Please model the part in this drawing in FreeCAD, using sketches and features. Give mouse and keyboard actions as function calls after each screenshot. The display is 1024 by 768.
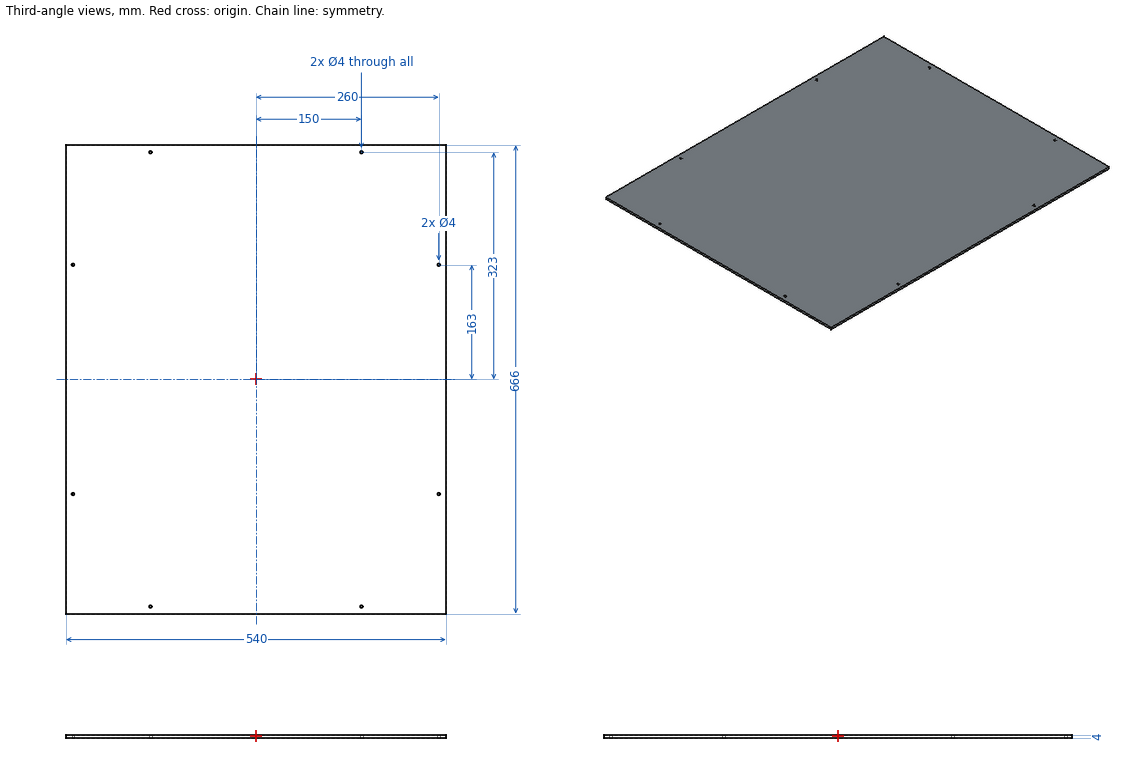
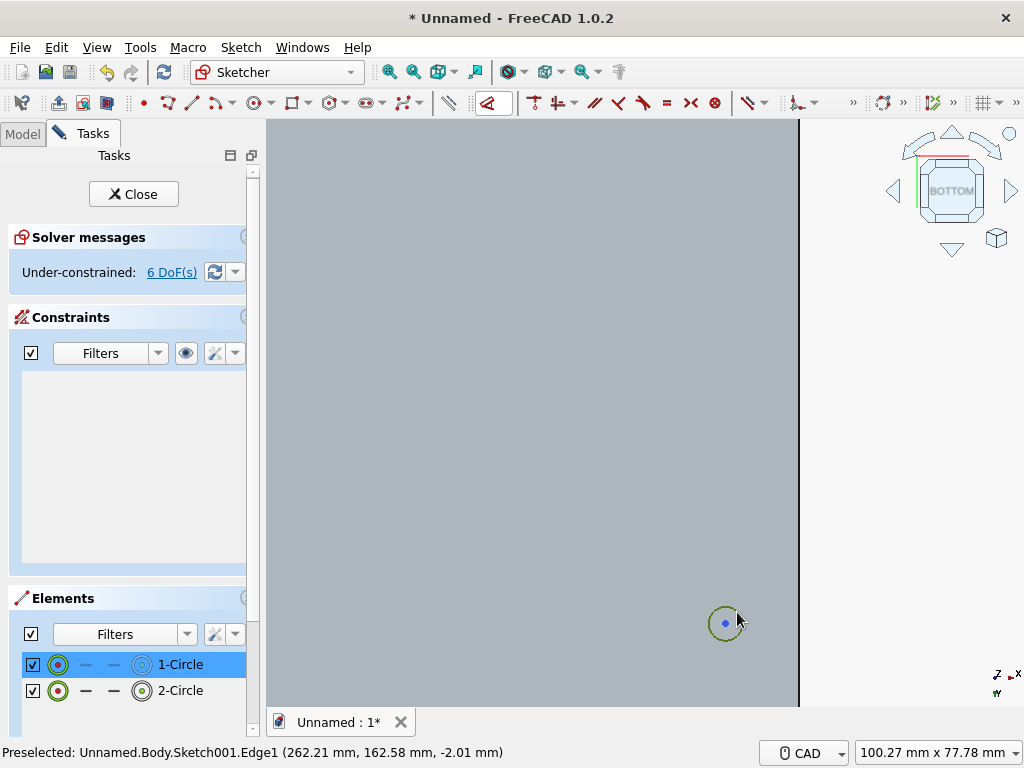
scroll(740, 616, down, 9)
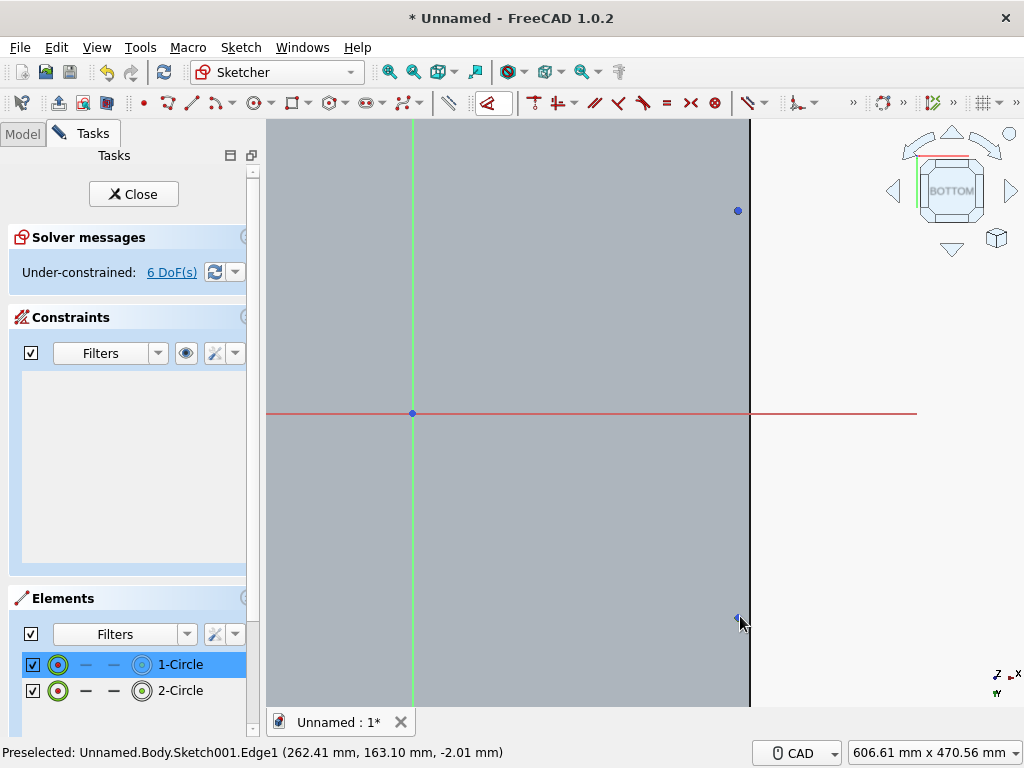
scroll(740, 209, up, 8)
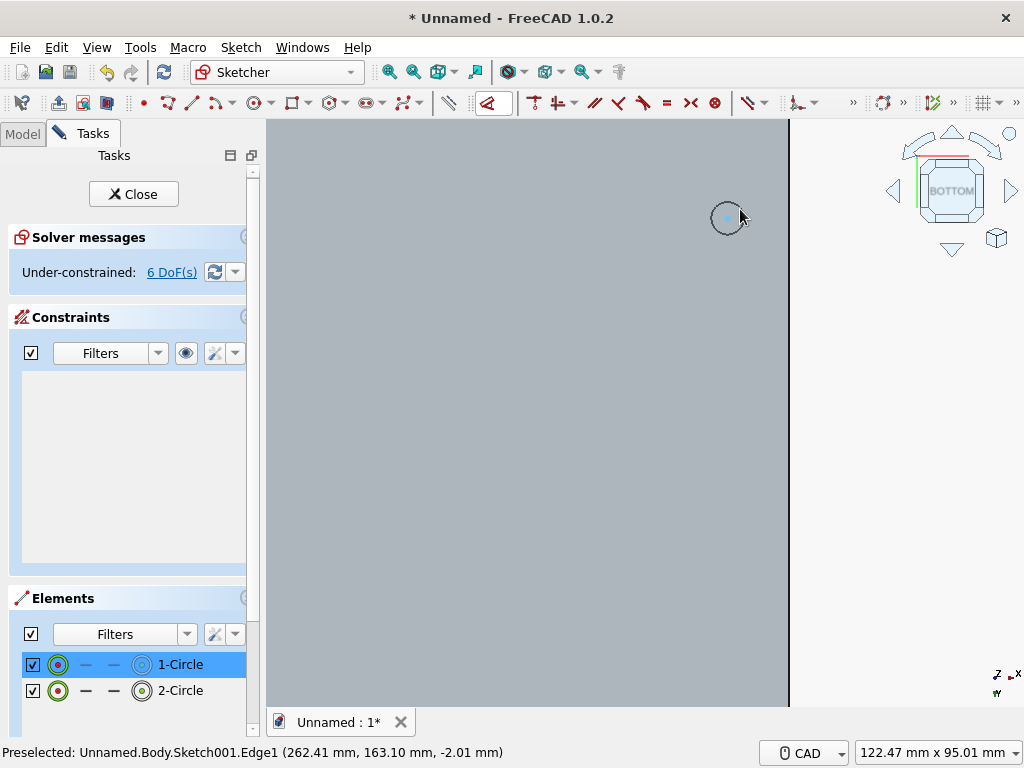
click(739, 207)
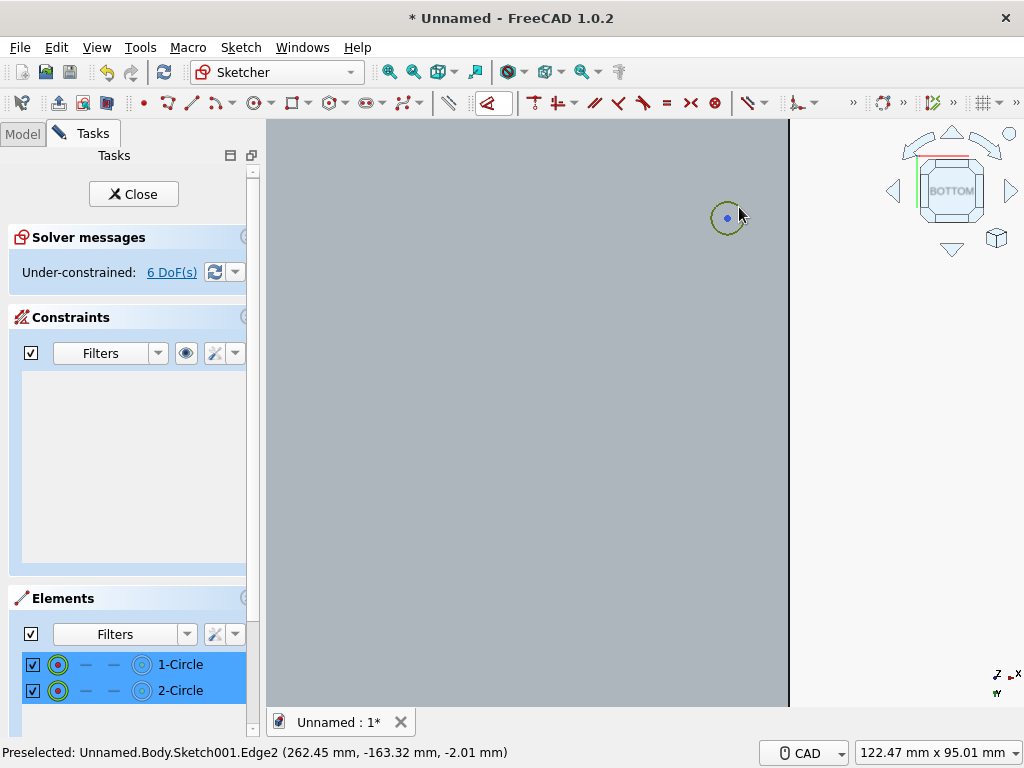
key(e)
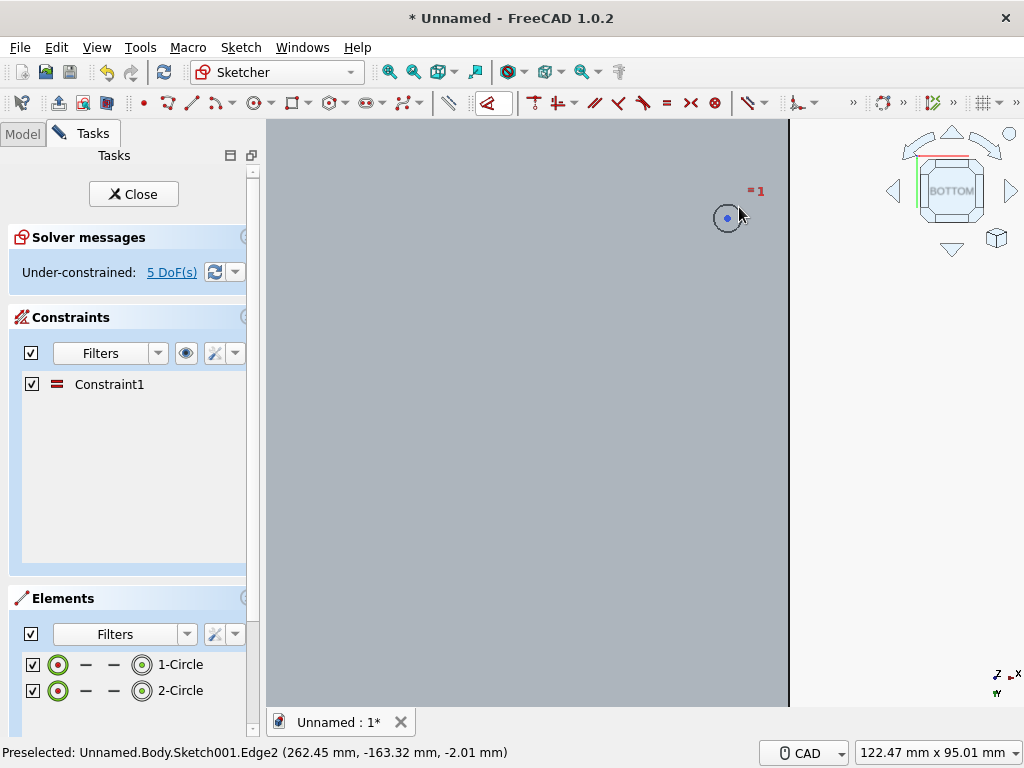
scroll(740, 209, down, 8)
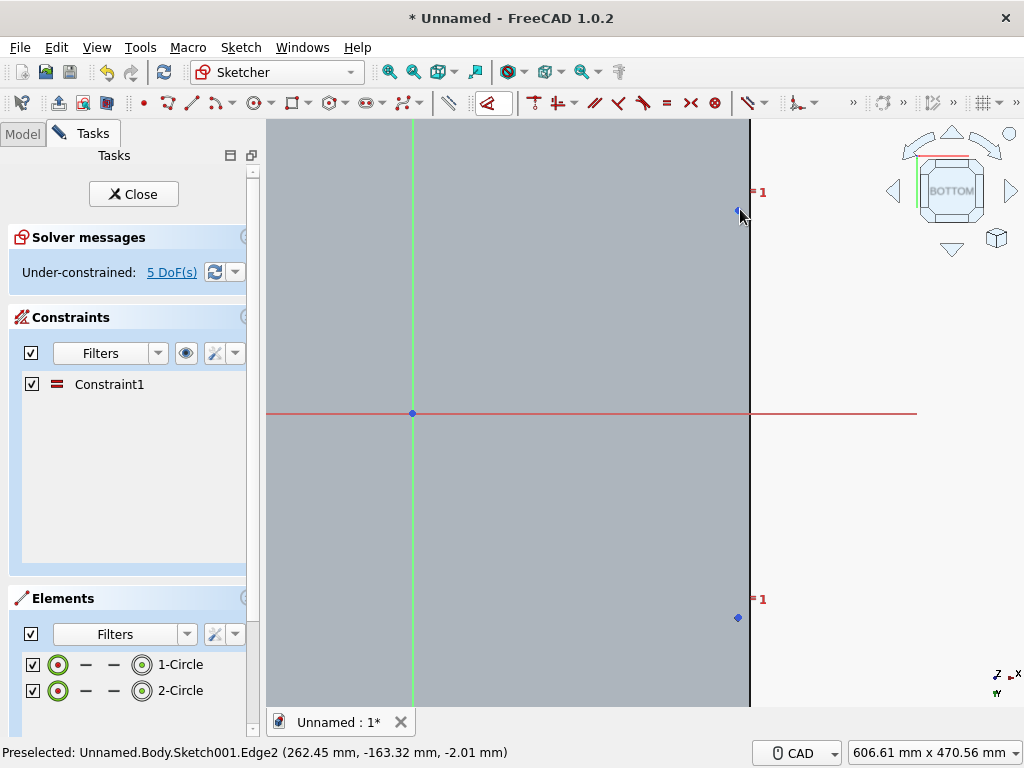
click(738, 618)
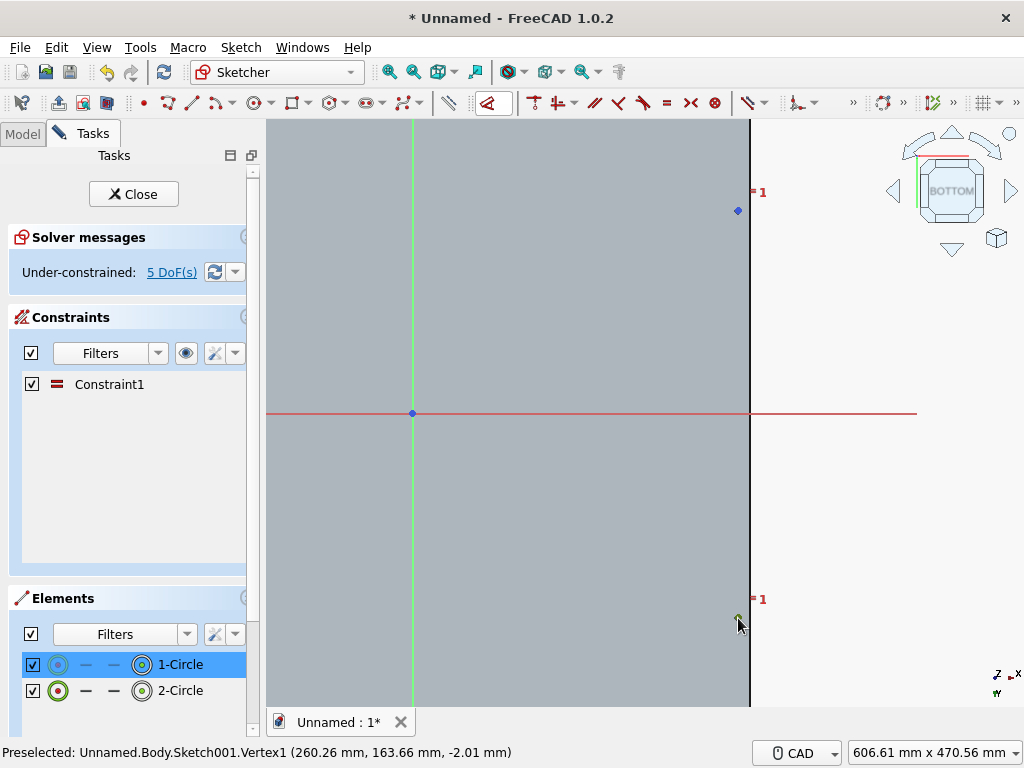
click(738, 211)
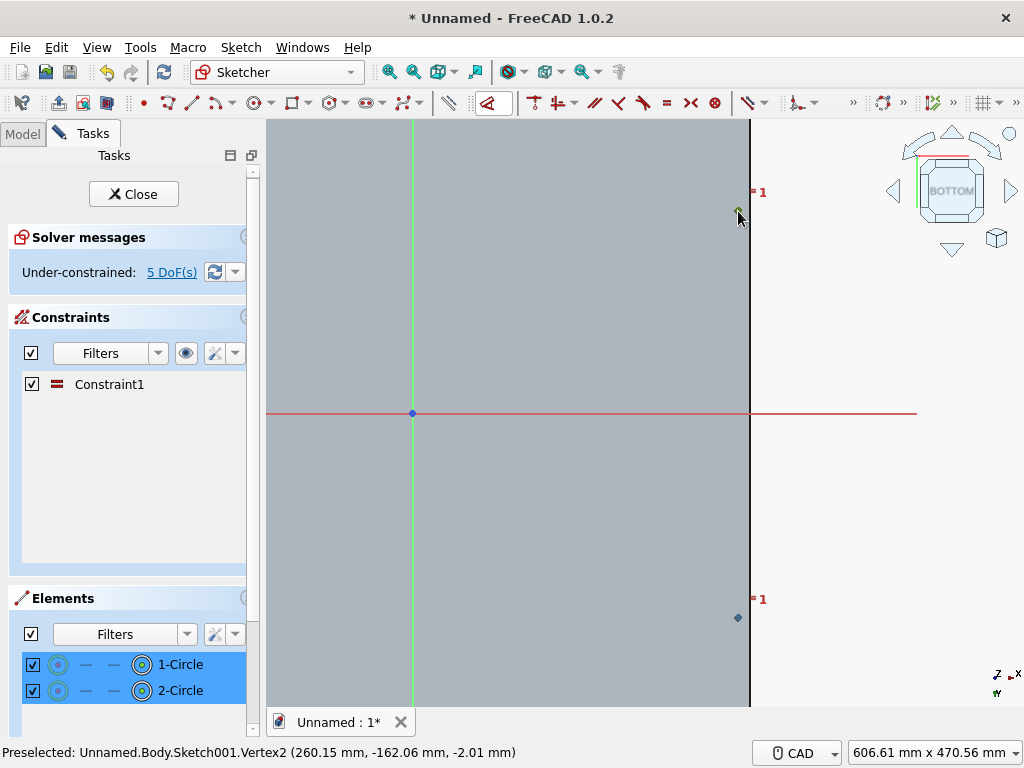
click(334, 413)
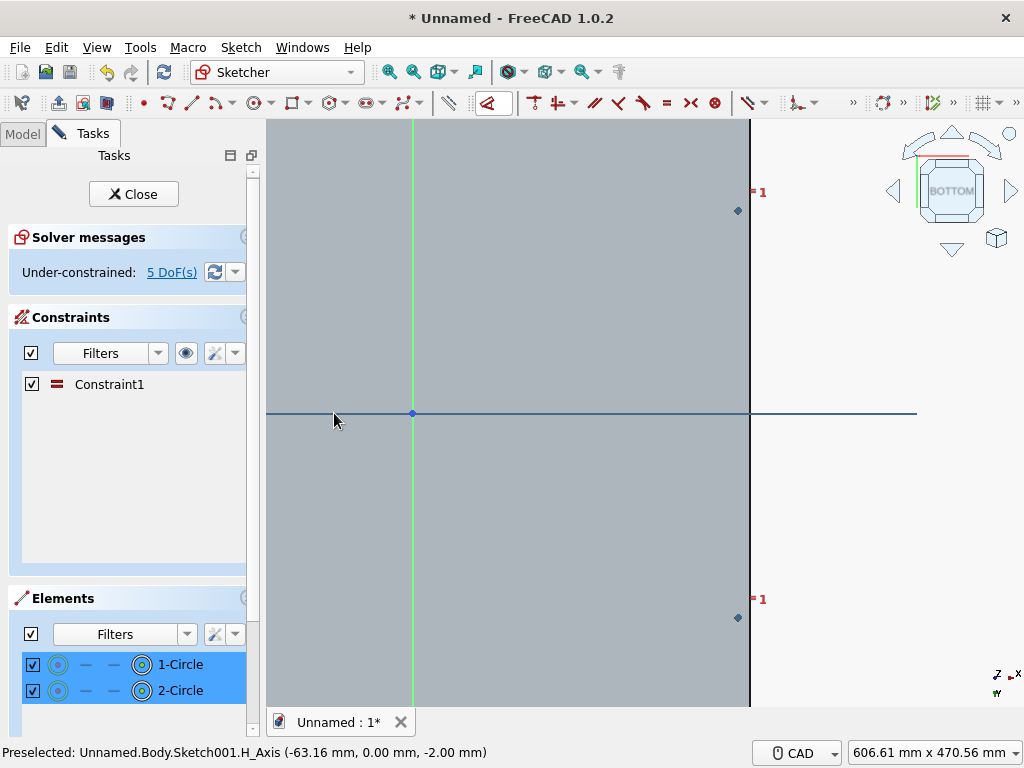
key(s)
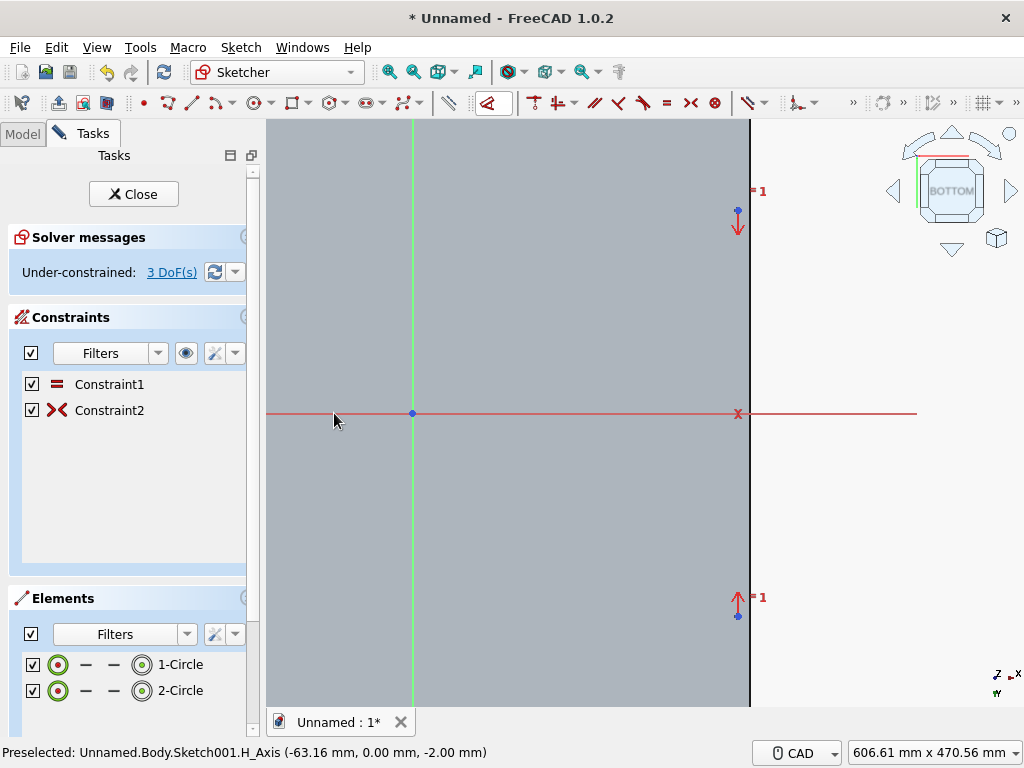
scroll(736, 615, up, 11)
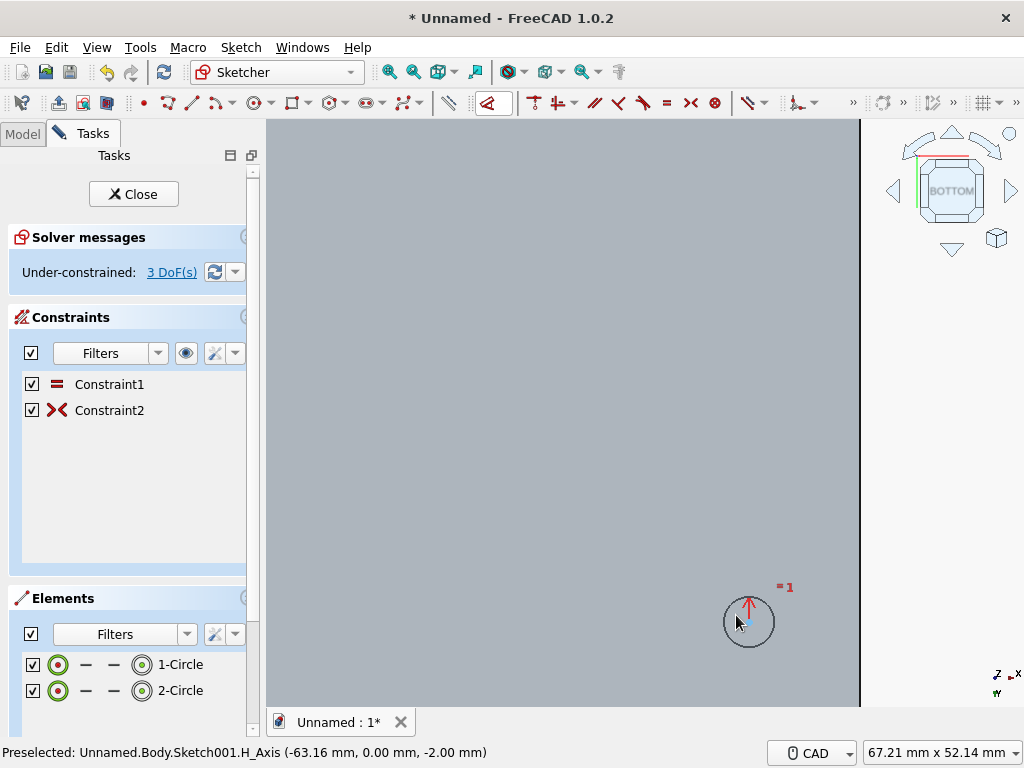
click(731, 604)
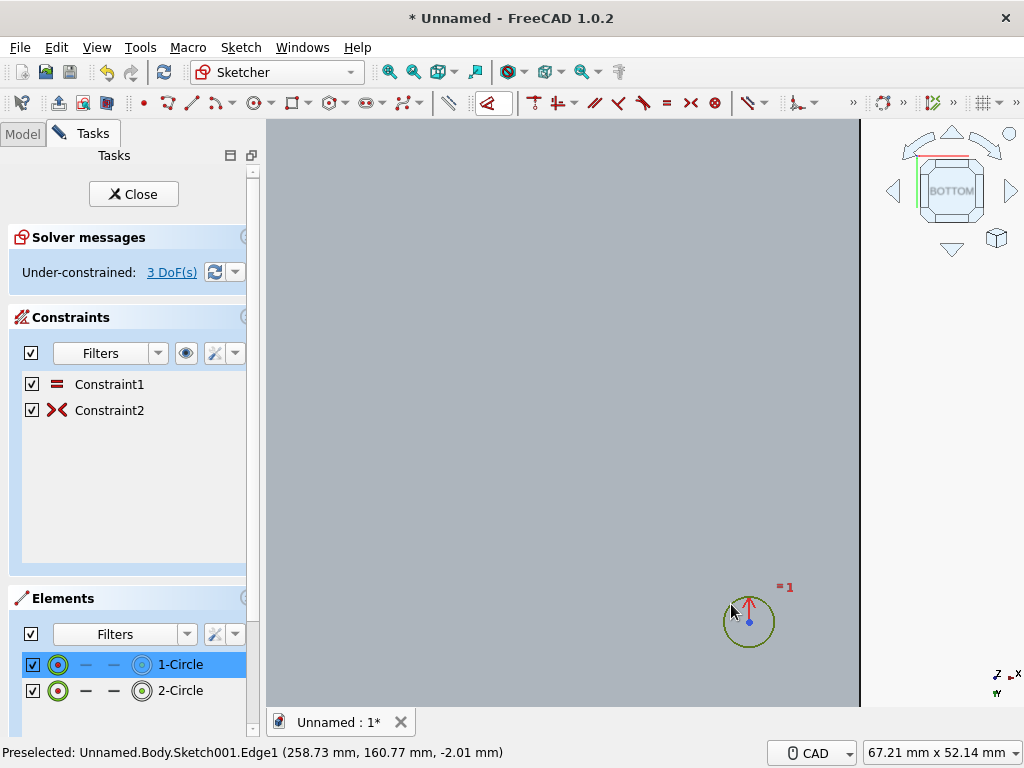
key(k)
key(o)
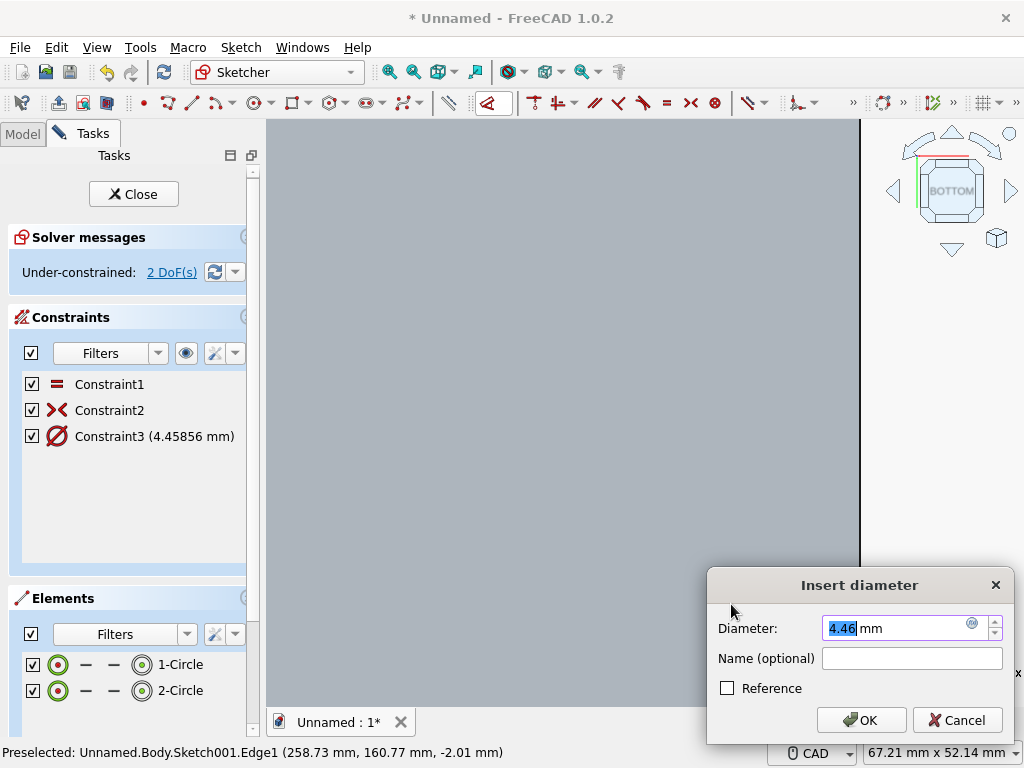
text(4)
key(Return)